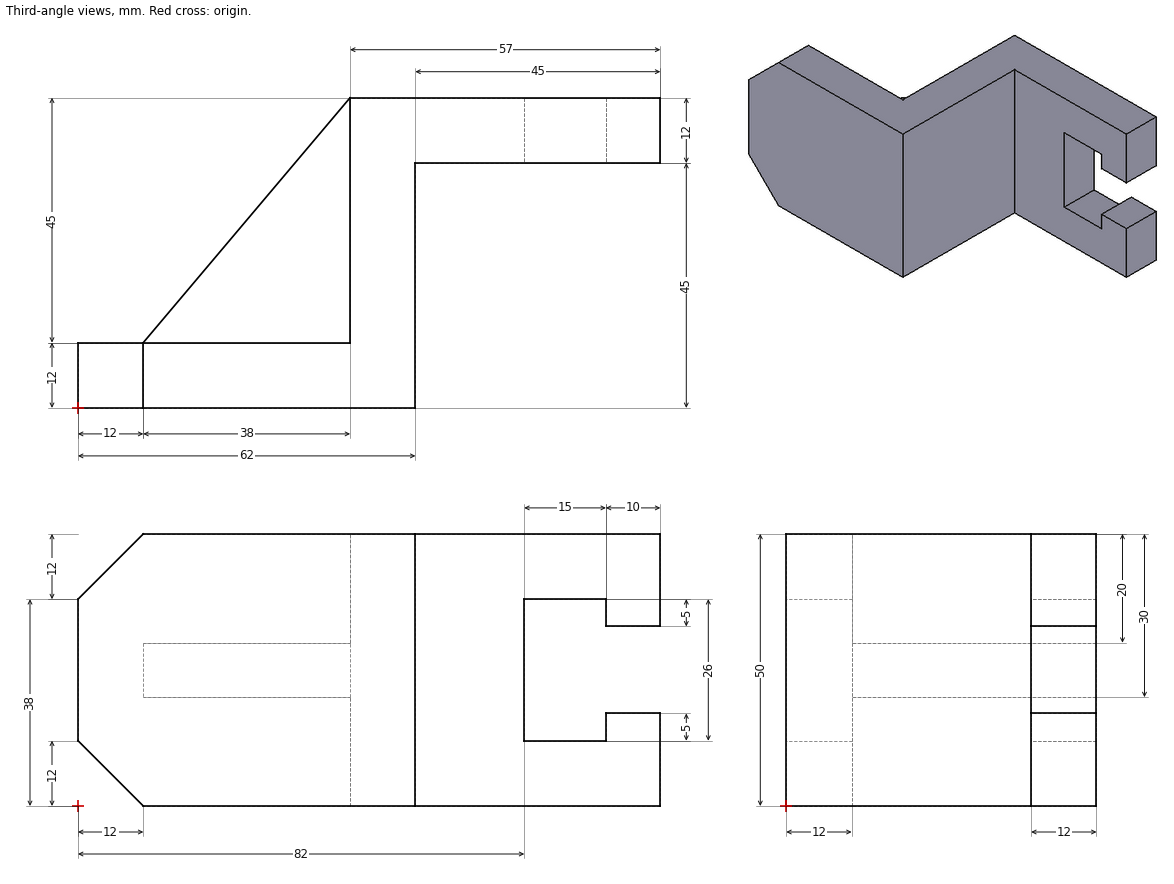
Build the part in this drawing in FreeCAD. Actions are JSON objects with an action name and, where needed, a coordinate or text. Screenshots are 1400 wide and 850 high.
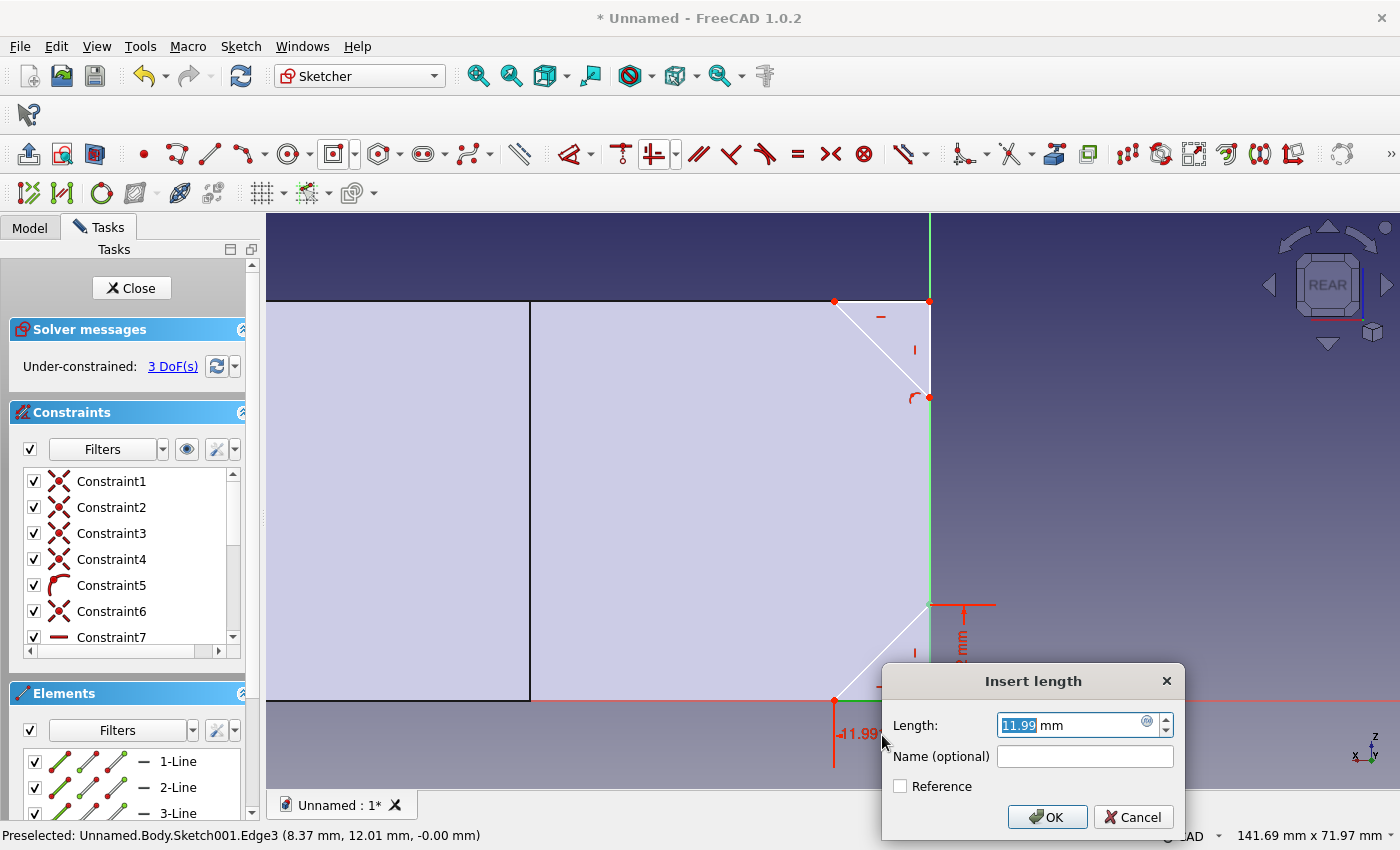
{"action": "type", "text": "12"}
{"action": "key", "text": "Return"}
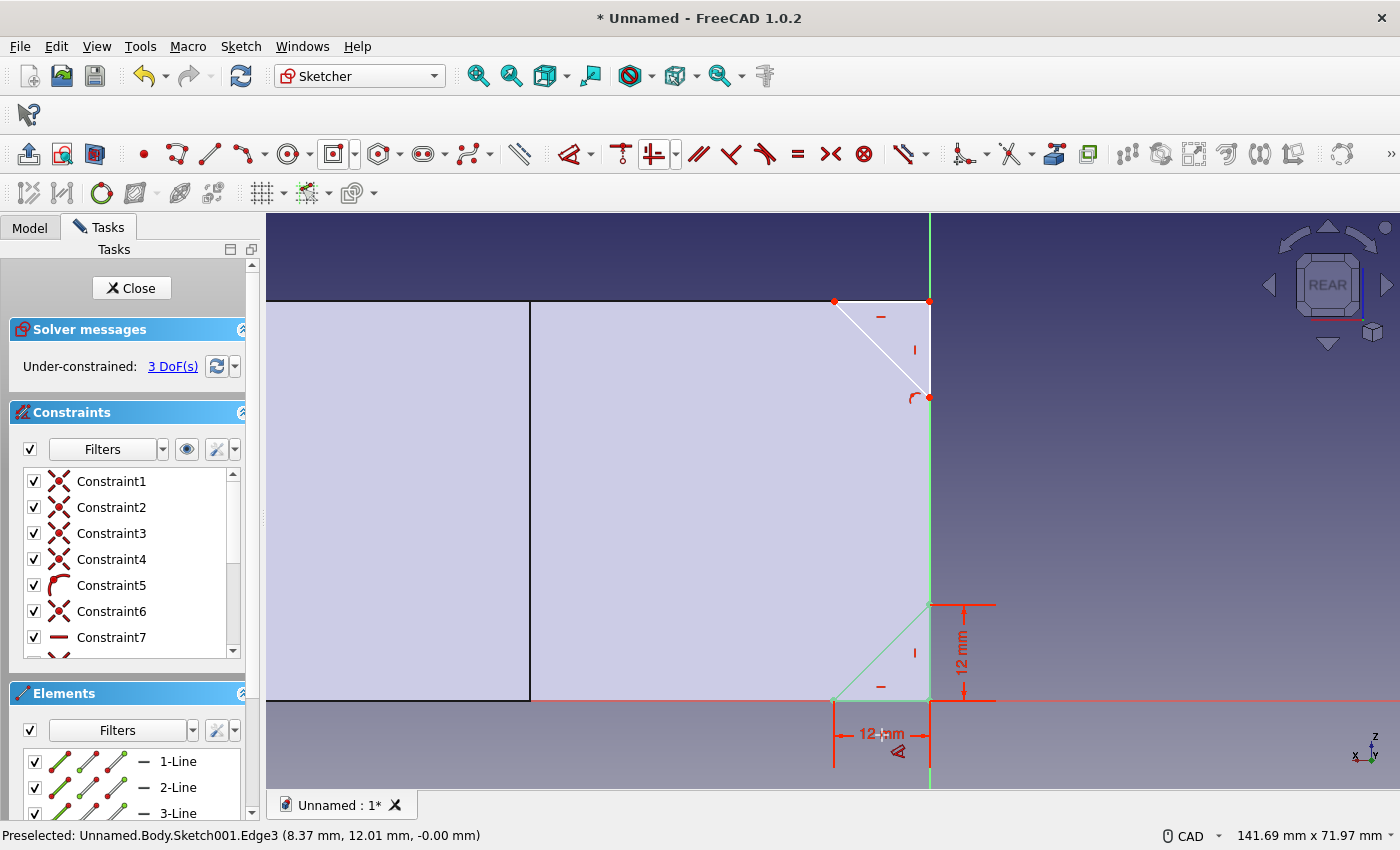
{"action": "left_click", "coordinate": [930, 369]}
{"action": "left_click", "coordinate": [964, 350]}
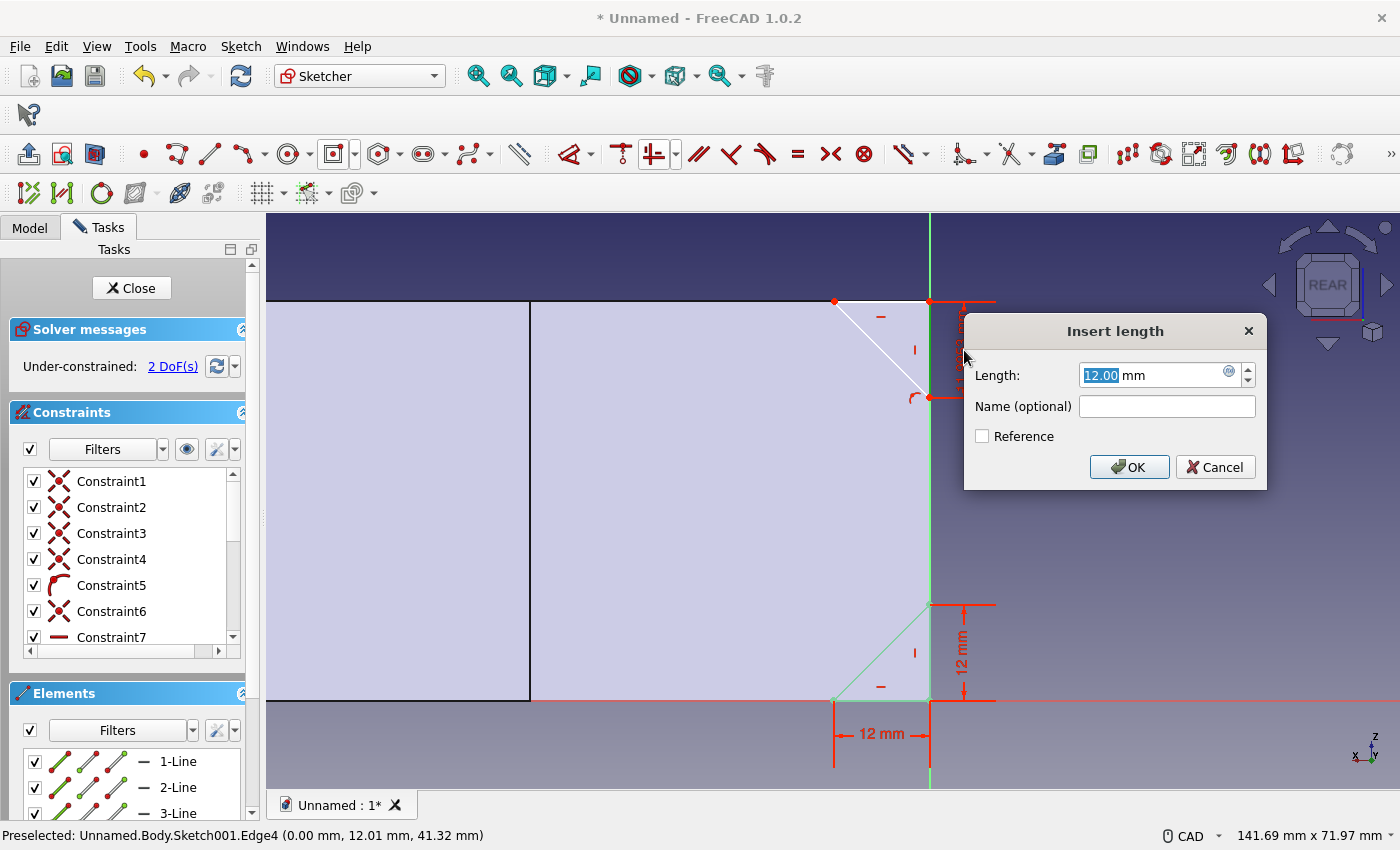
{"action": "type", "text": "12"}
{"action": "key", "text": "Return"}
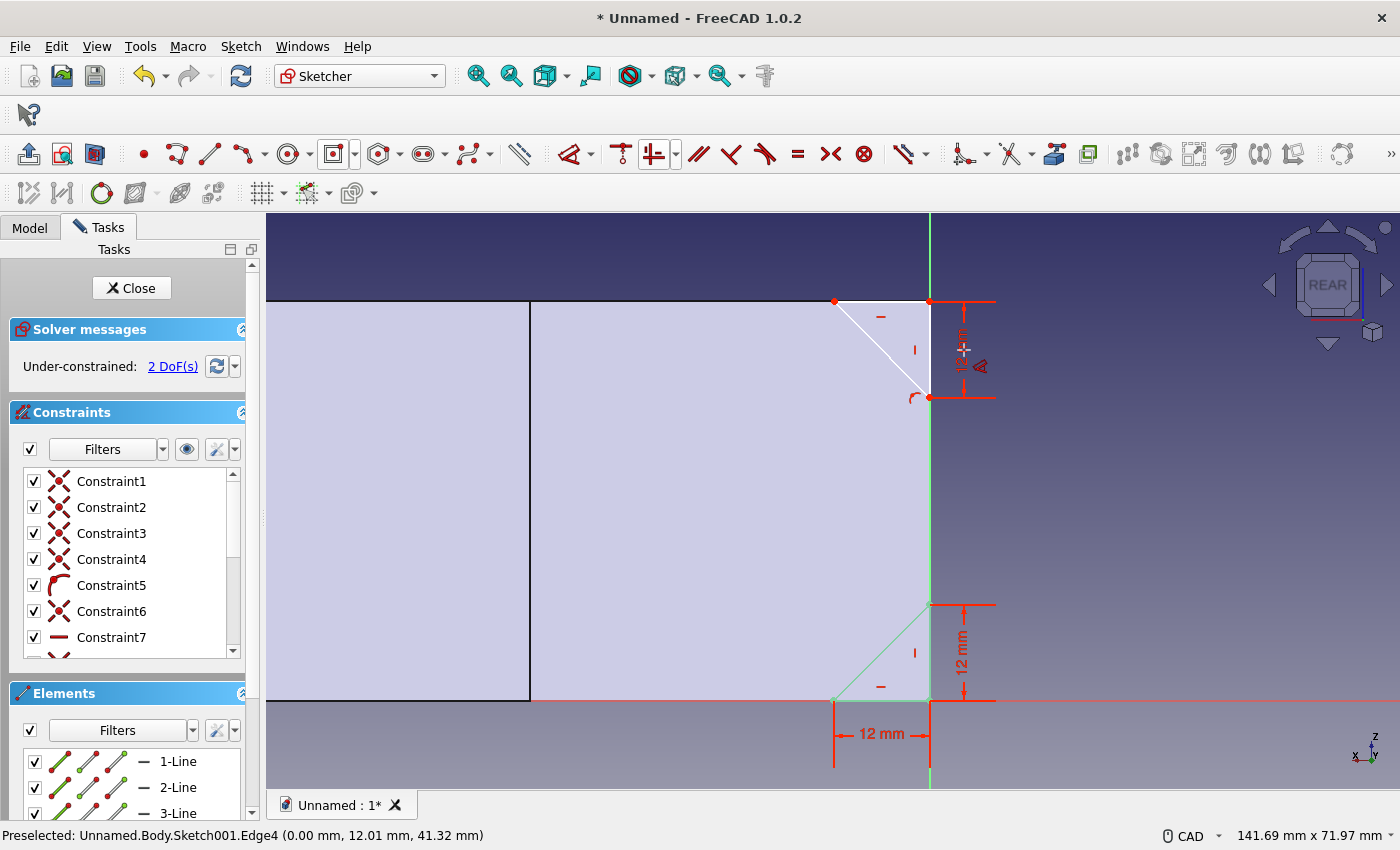
{"action": "left_click", "coordinate": [901, 302]}
{"action": "left_click", "coordinate": [882, 268]}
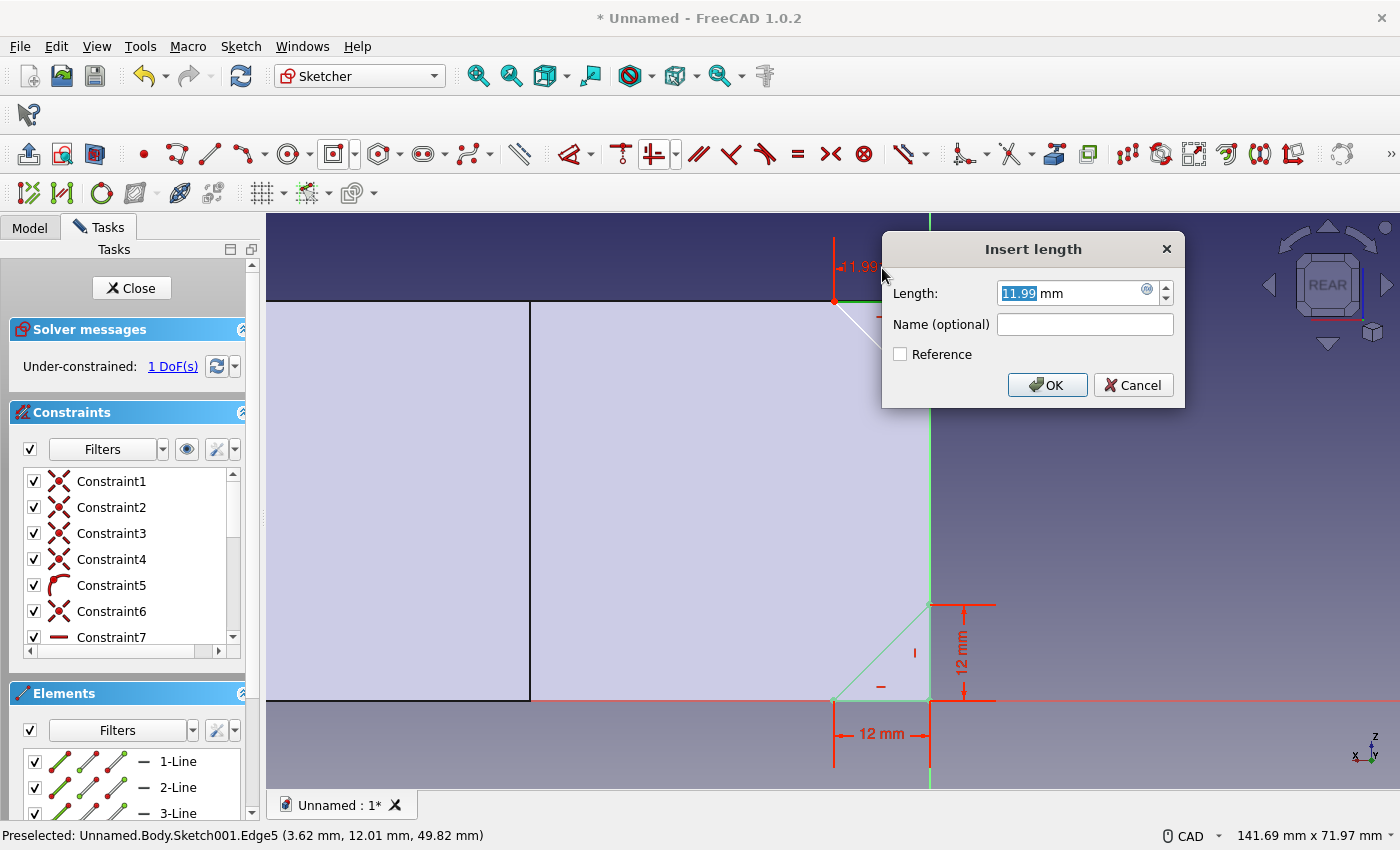
{"action": "type", "text": "12"}
{"action": "key", "text": "Return"}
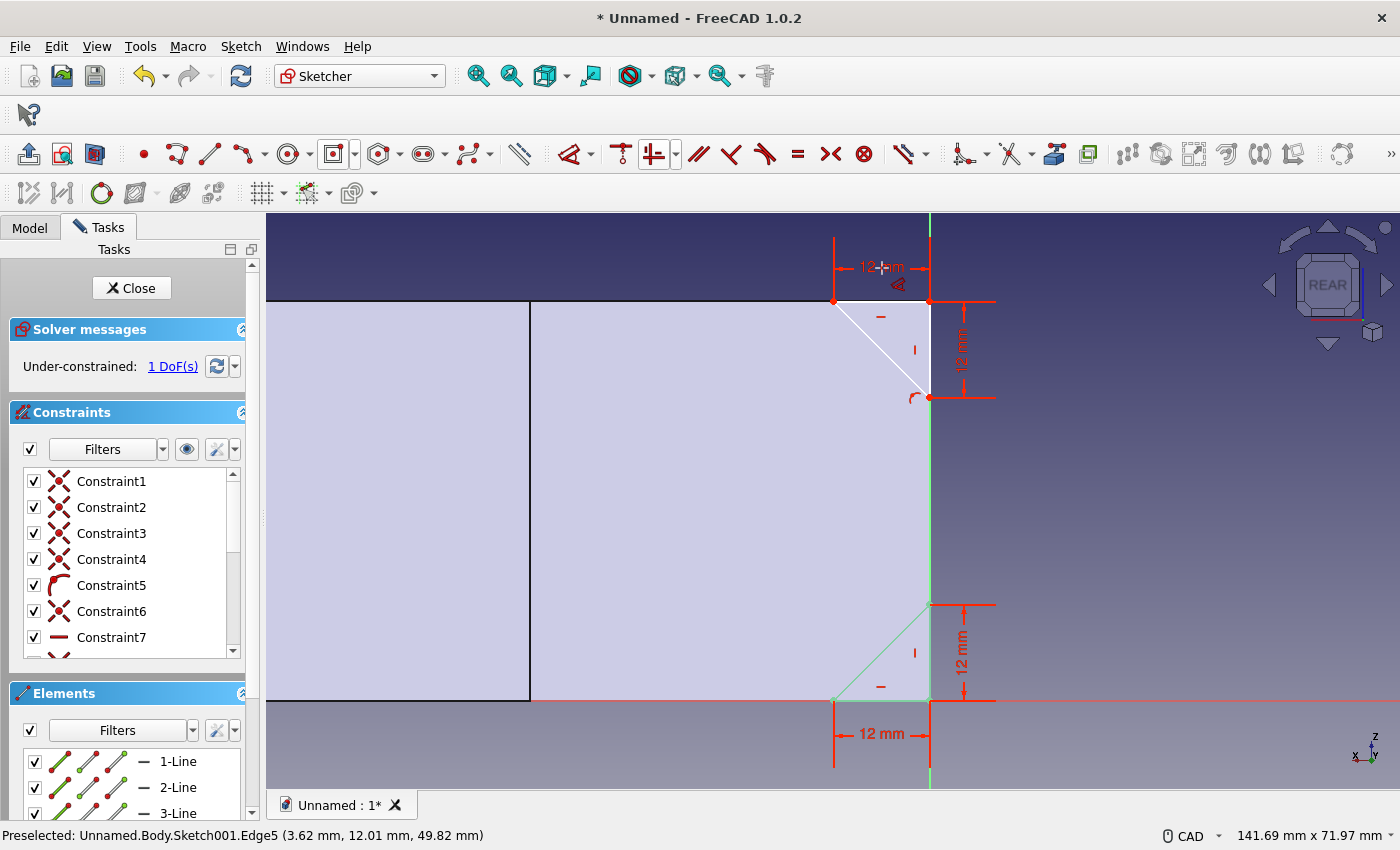
{"action": "left_click", "coordinate": [930, 398]}
{"action": "left_click", "coordinate": [964, 549]}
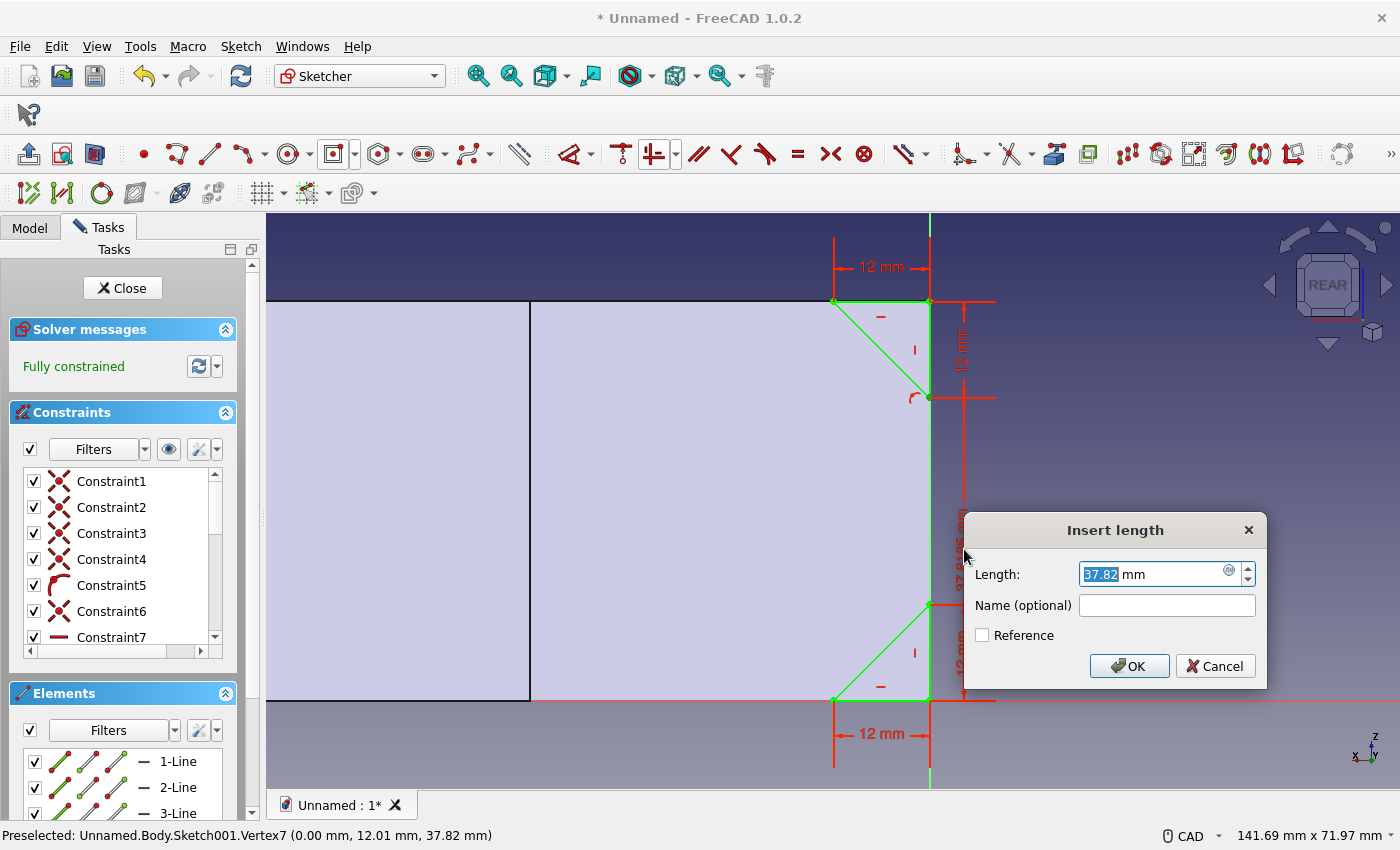
{"action": "type", "text": "38"}
{"action": "key", "text": "Return"}
{"action": "key", "text": "Escape"}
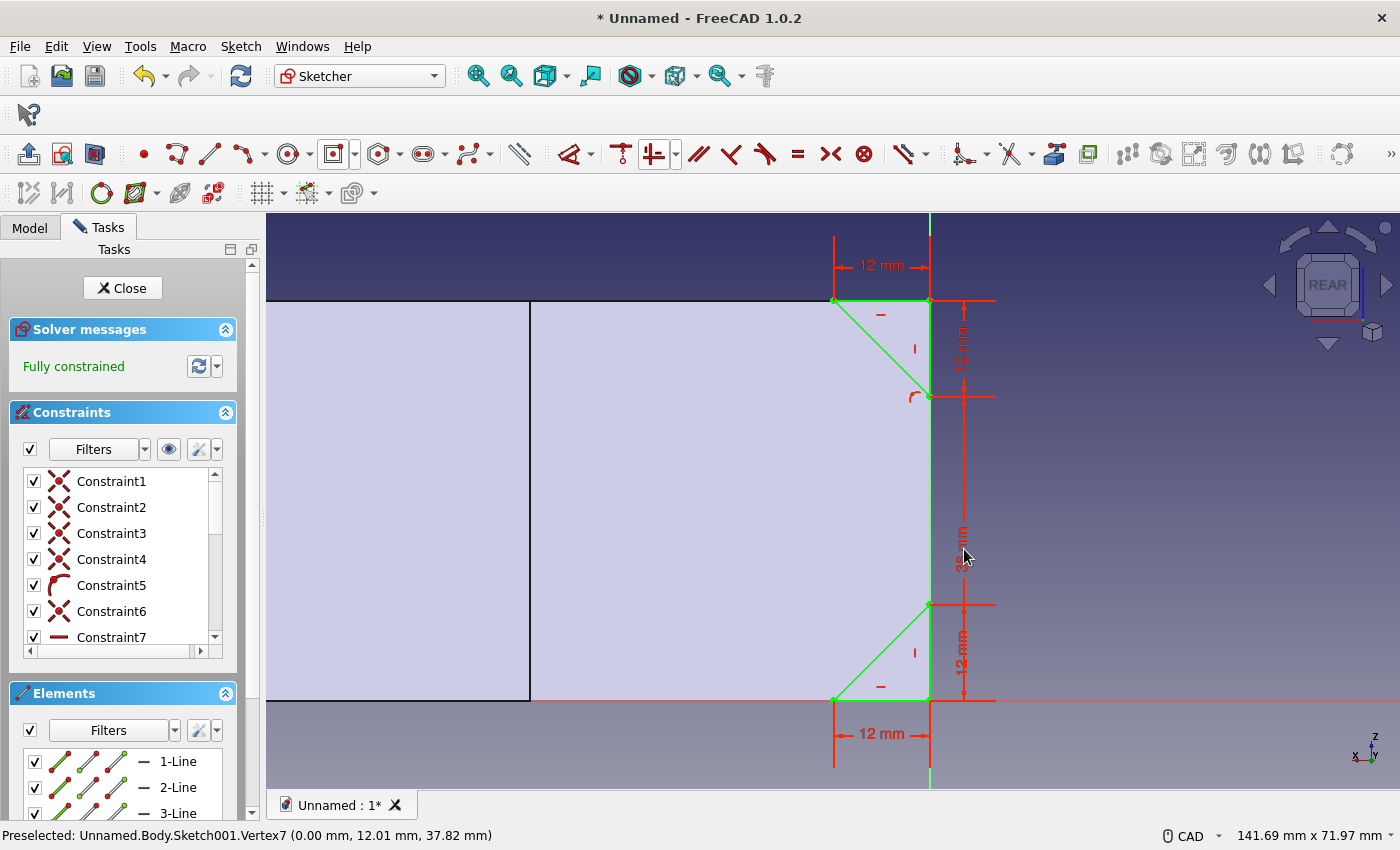
{"action": "left_click", "coordinate": [123, 288]}